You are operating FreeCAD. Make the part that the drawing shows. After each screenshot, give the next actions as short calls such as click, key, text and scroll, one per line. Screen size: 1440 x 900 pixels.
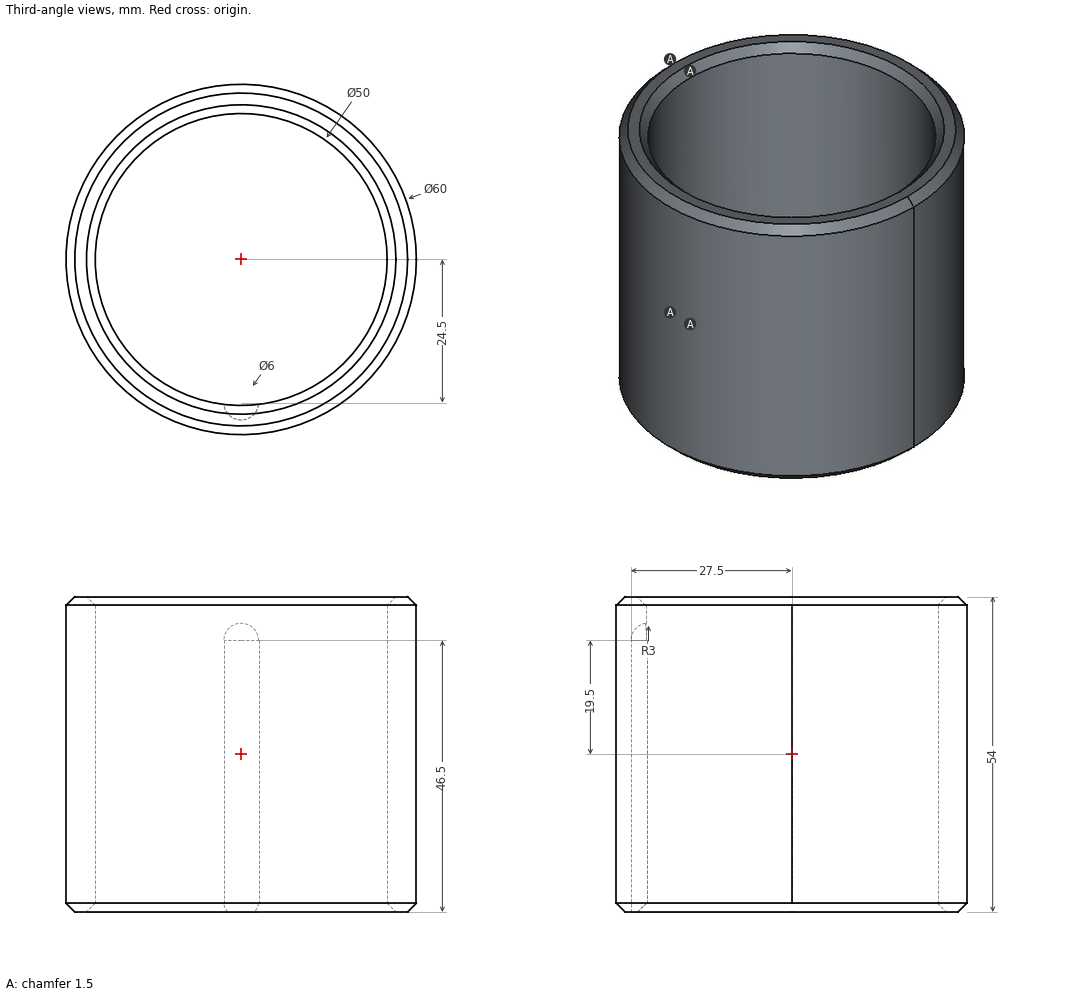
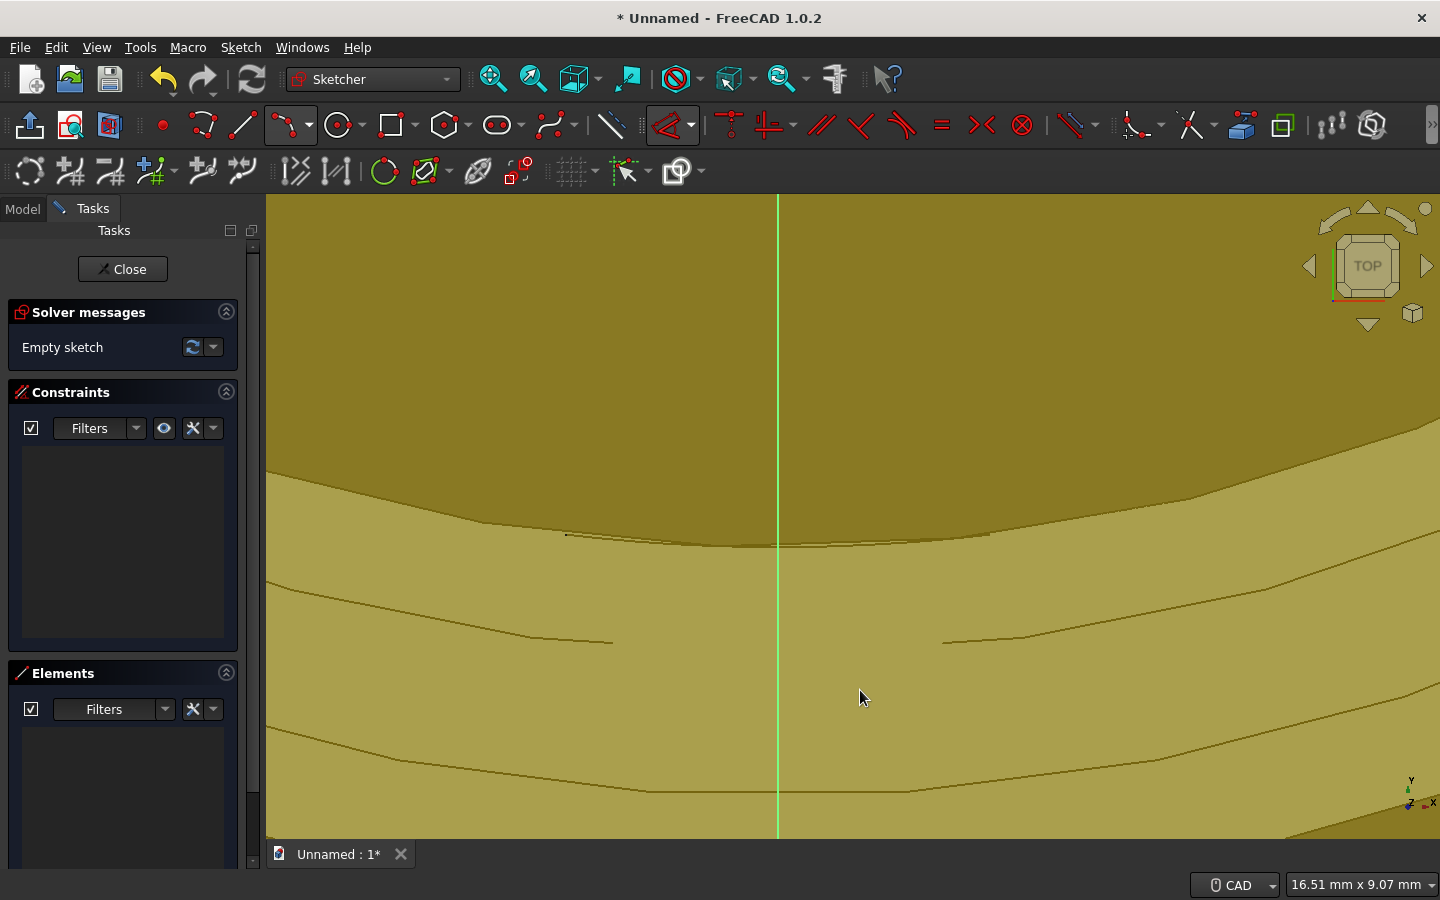
click(338, 126)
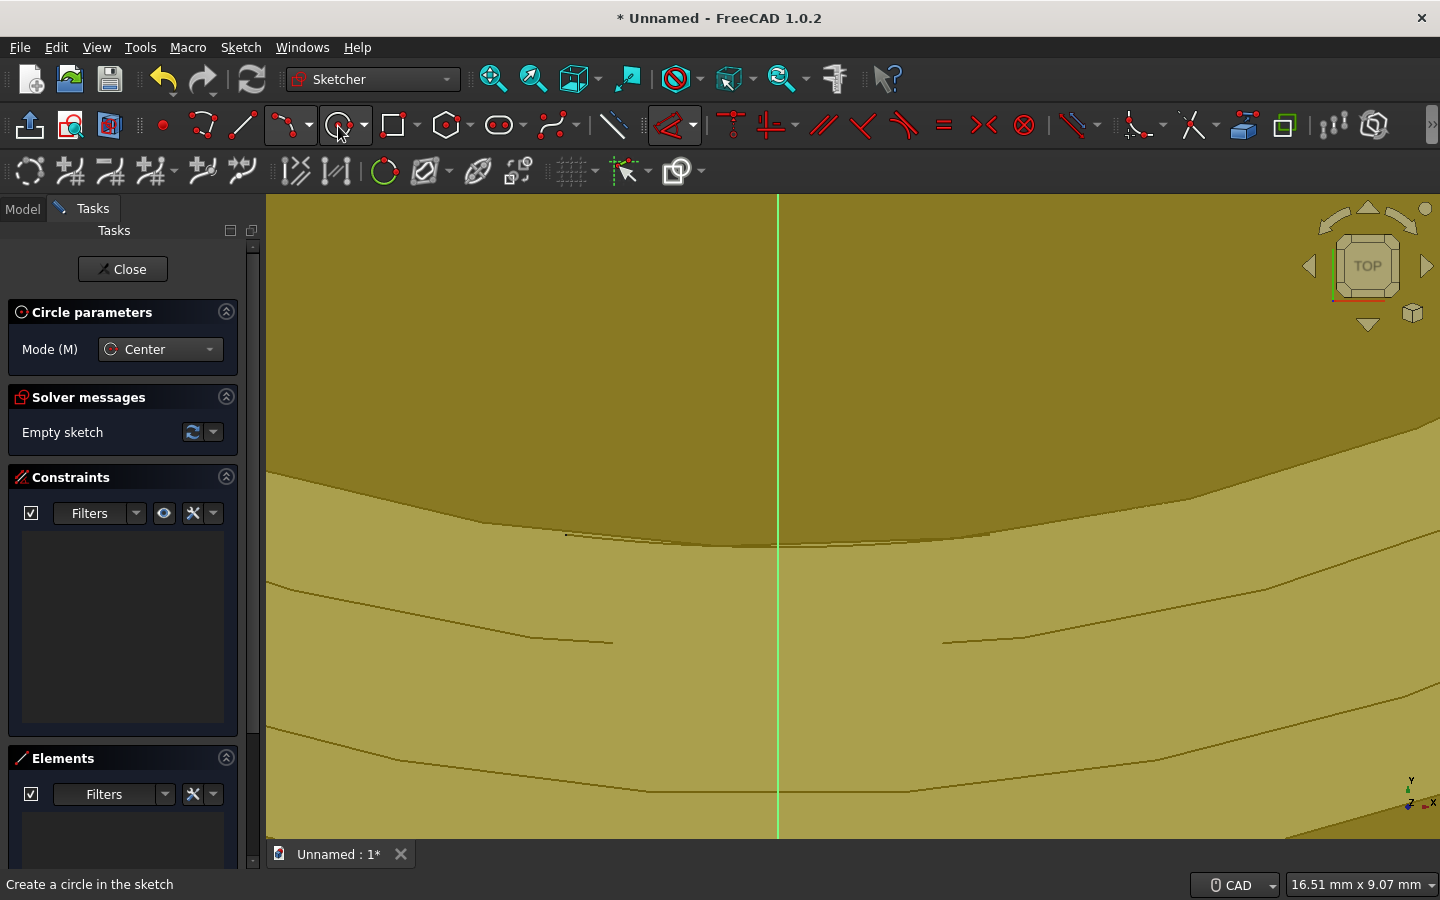
click(778, 512)
click(929, 361)
key(Escape)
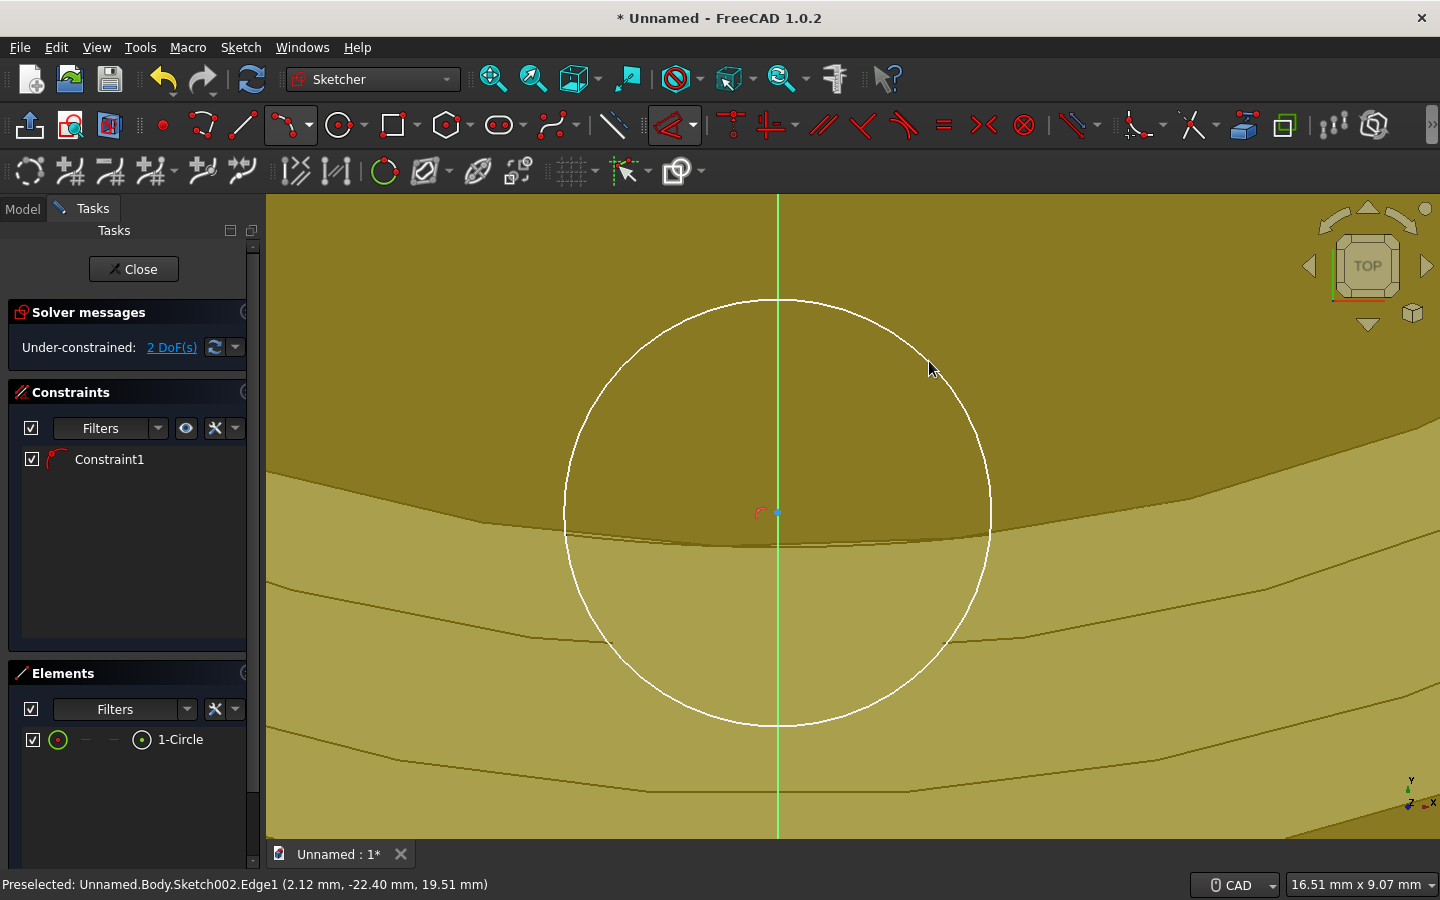
click(928, 361)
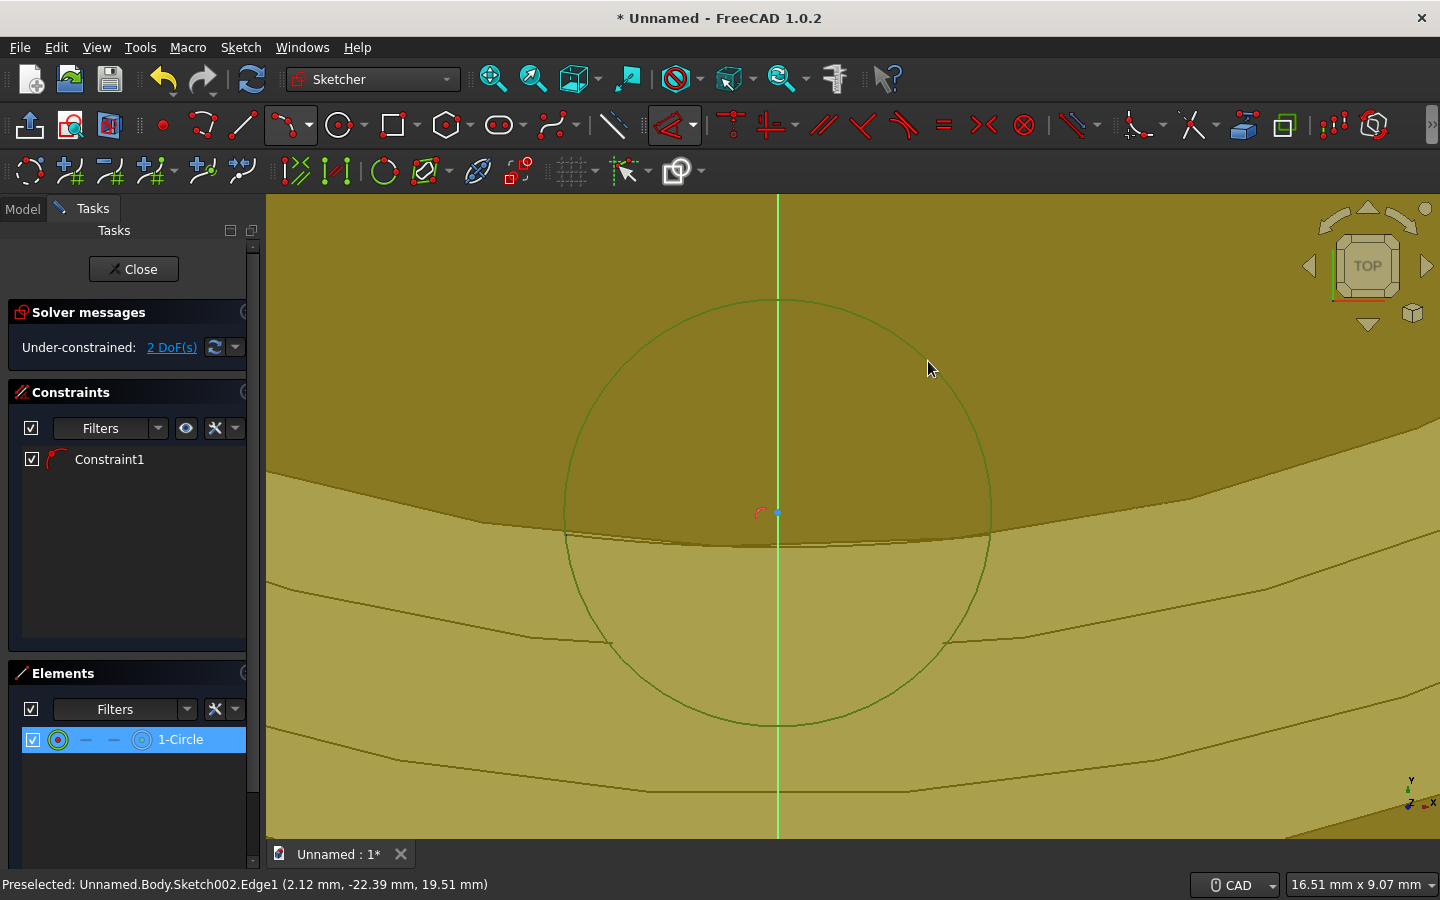
key(k)
key(o)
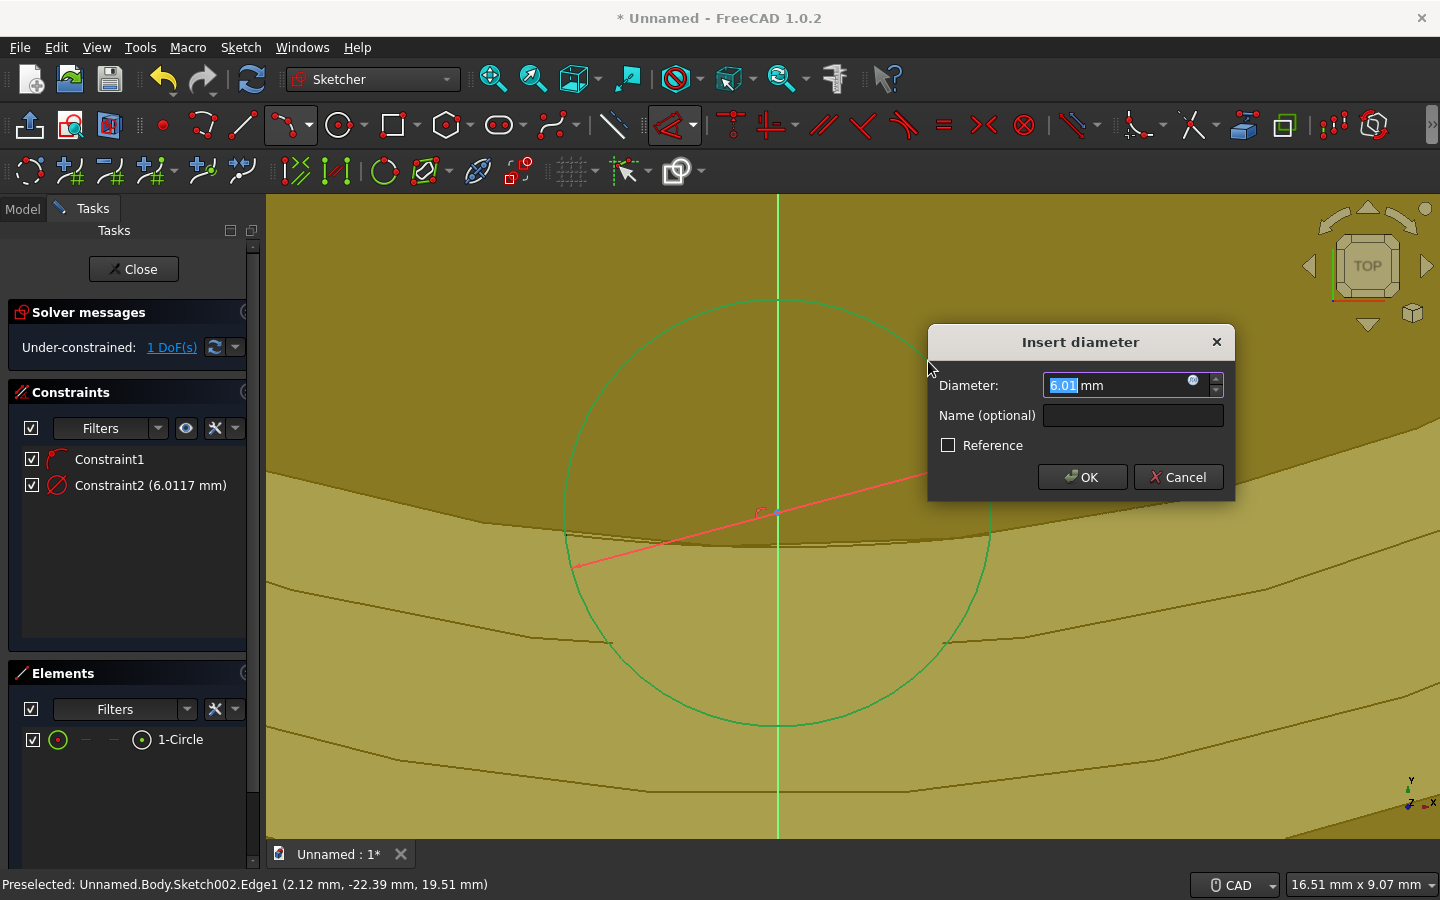
text(6)
key(Return)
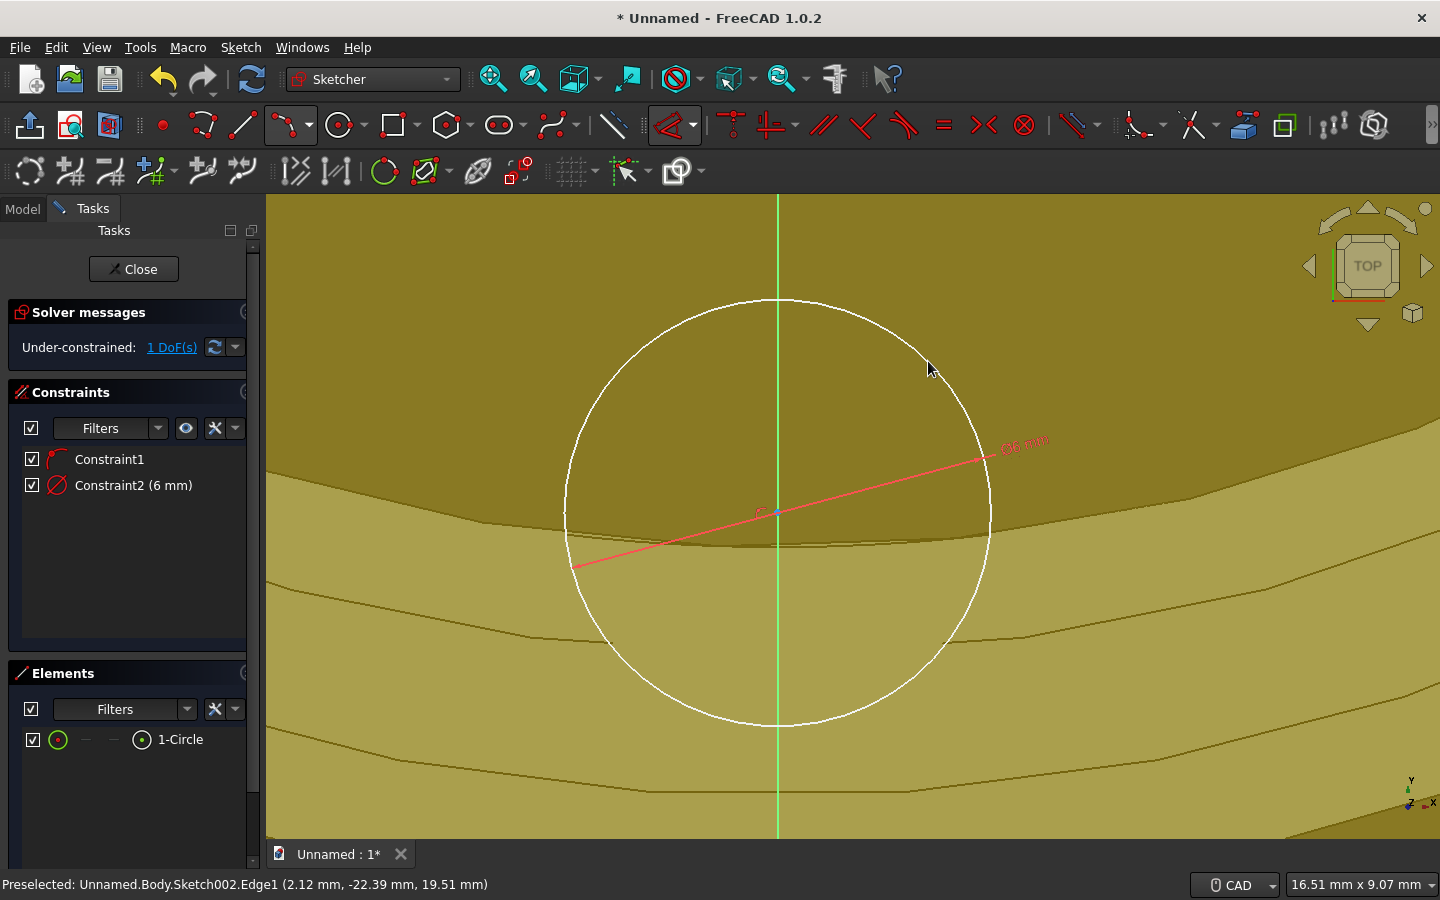
click(778, 513)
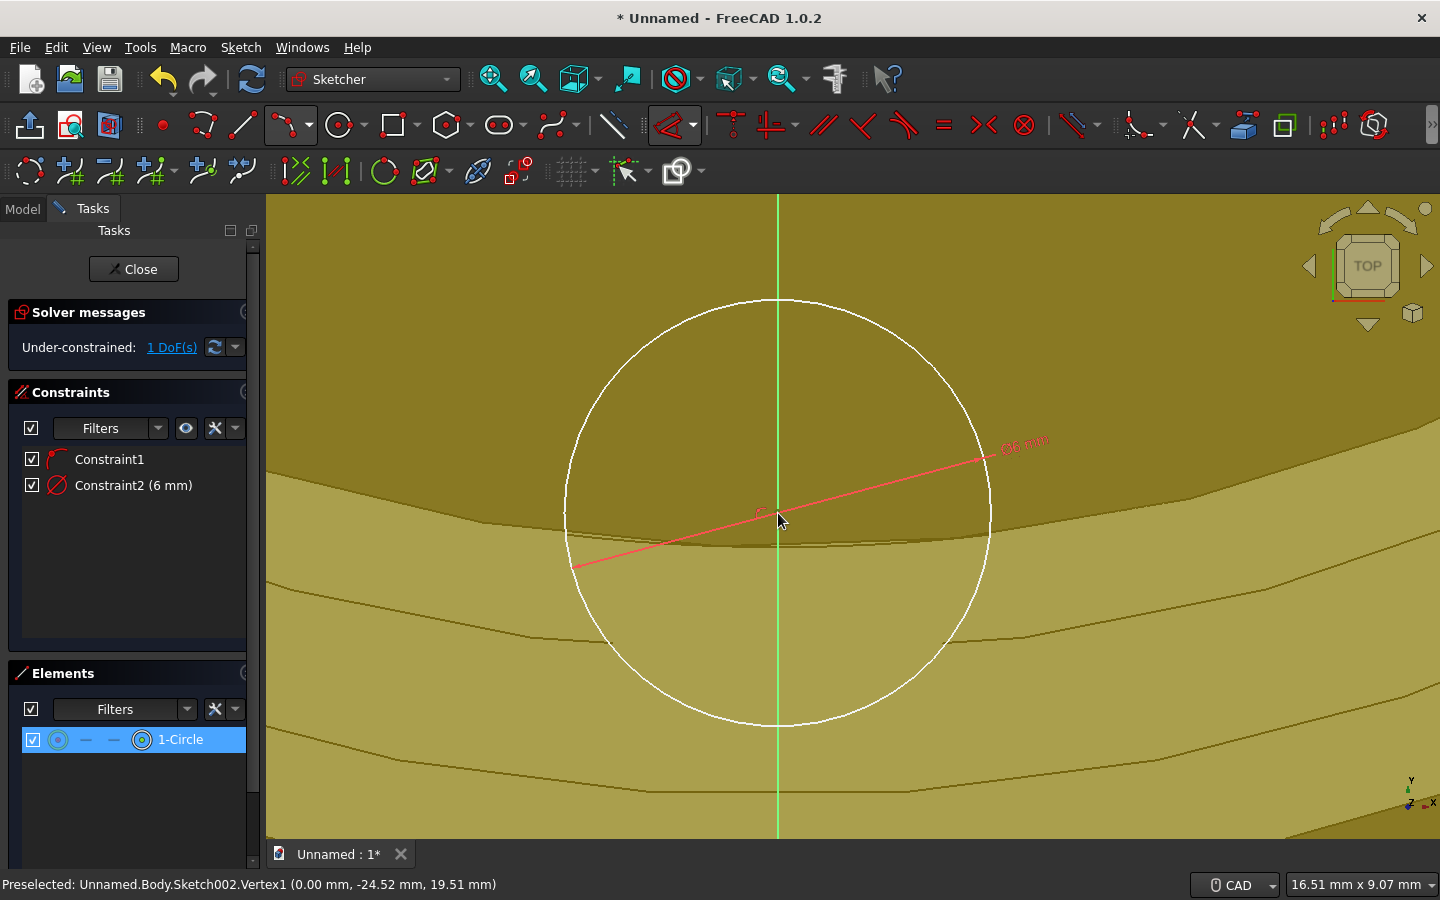
key(i)